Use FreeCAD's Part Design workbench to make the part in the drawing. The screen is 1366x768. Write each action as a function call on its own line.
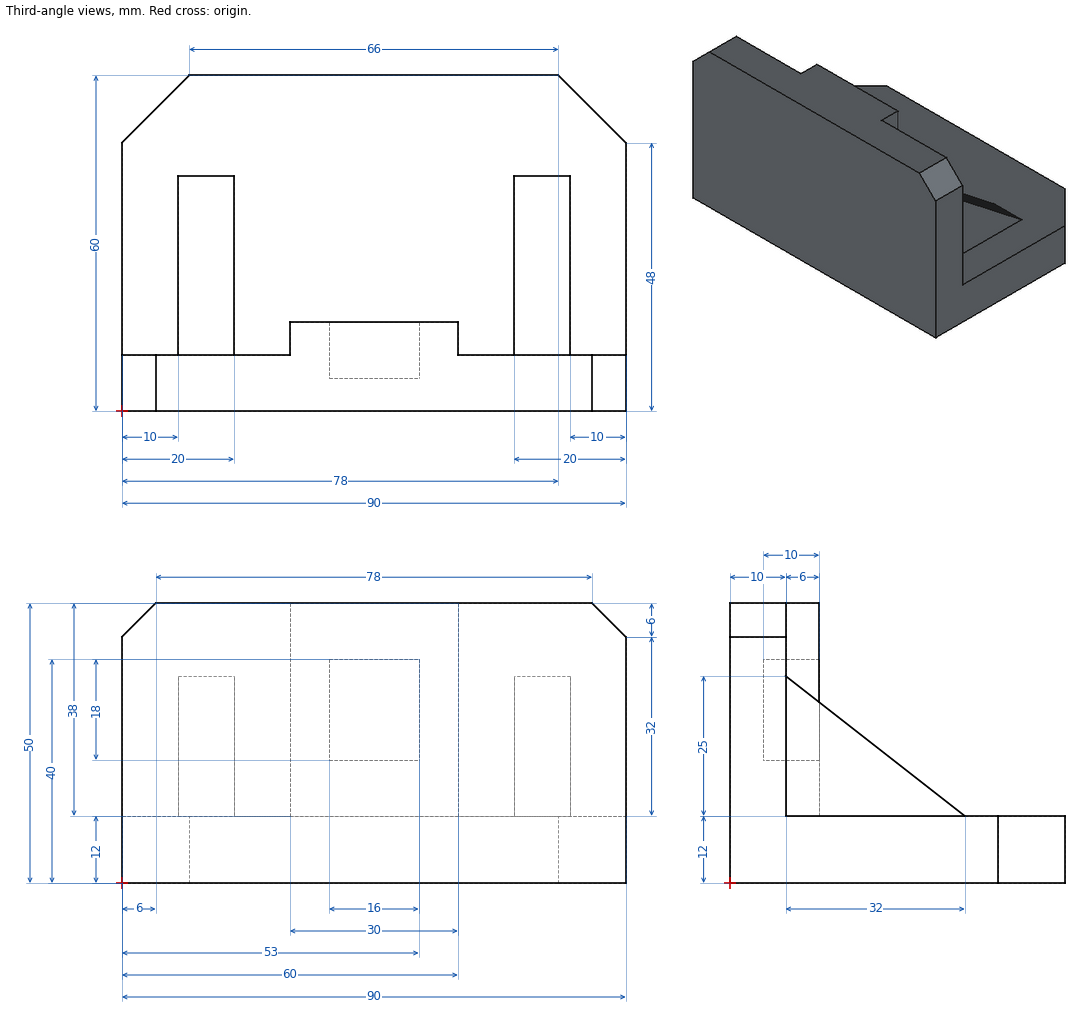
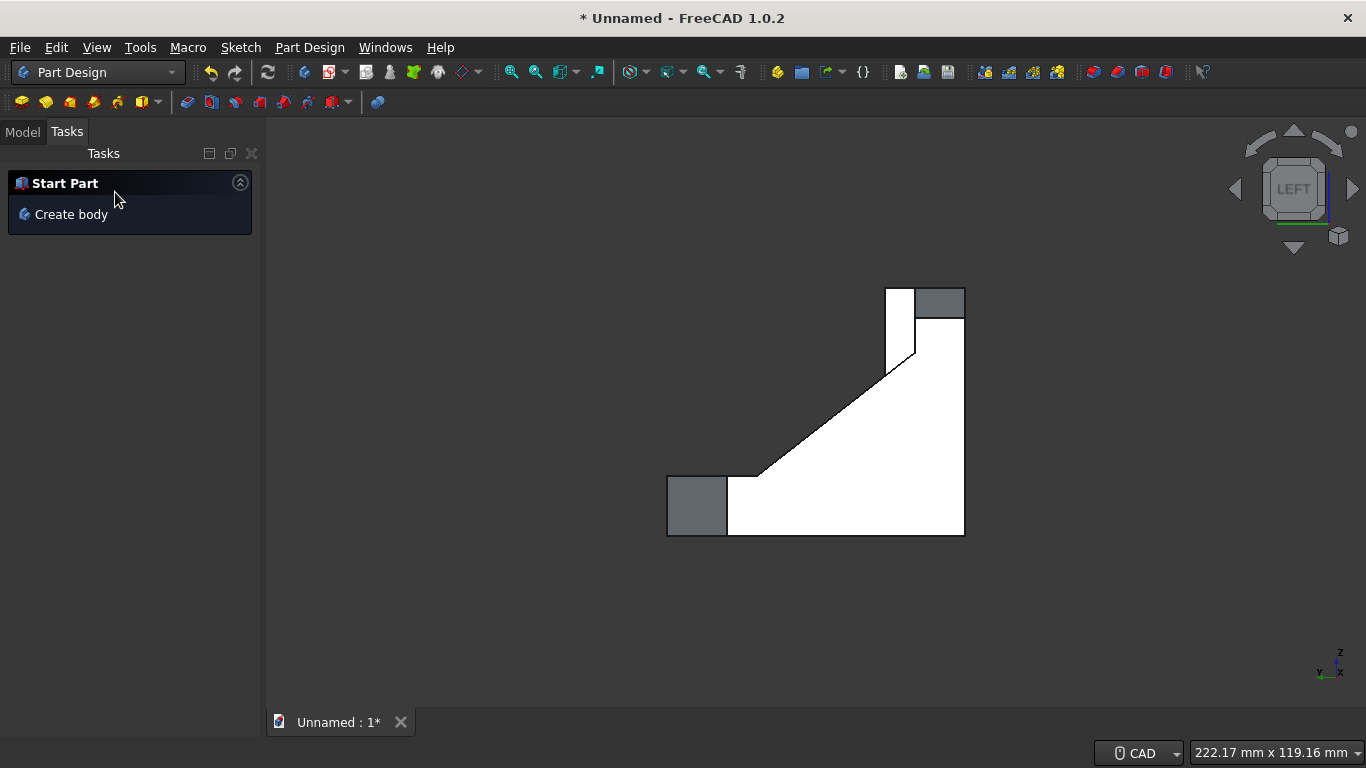
click(512, 72)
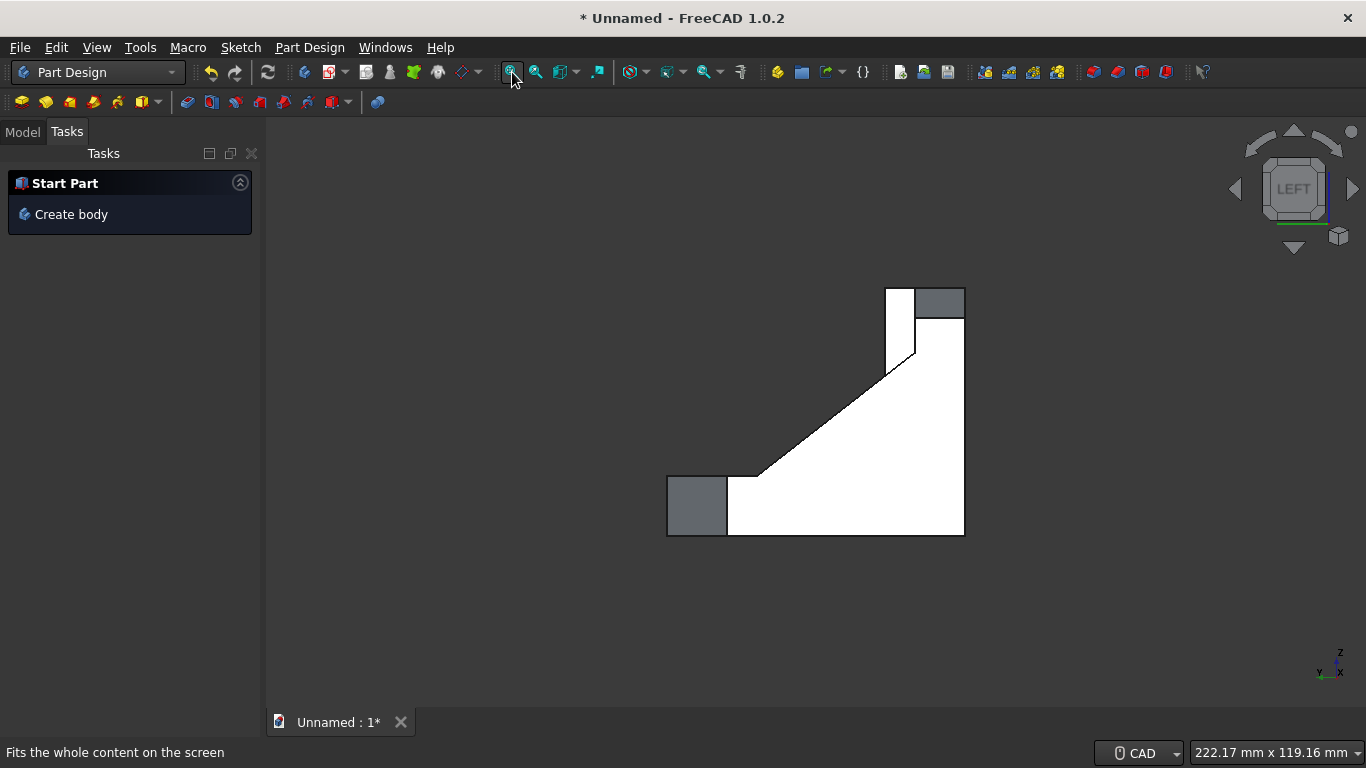
click(880, 457)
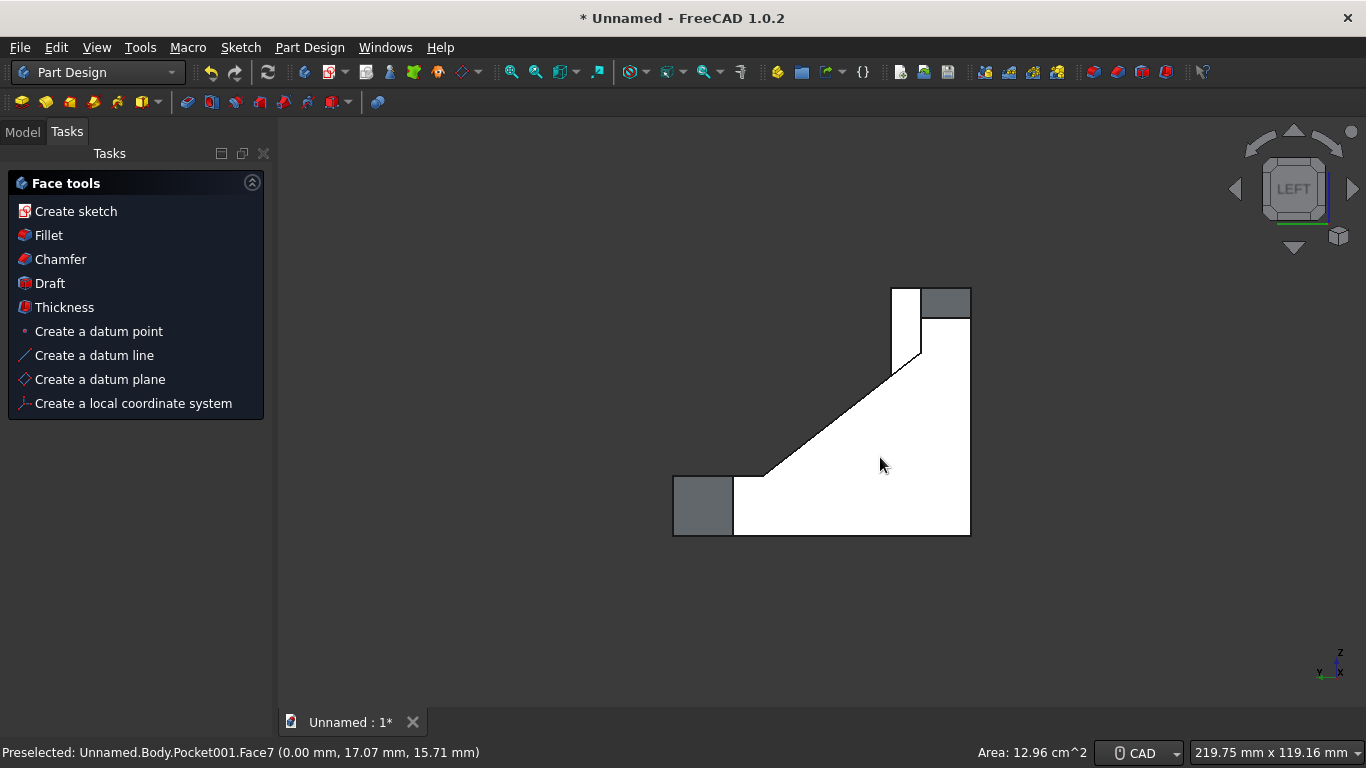
click(330, 72)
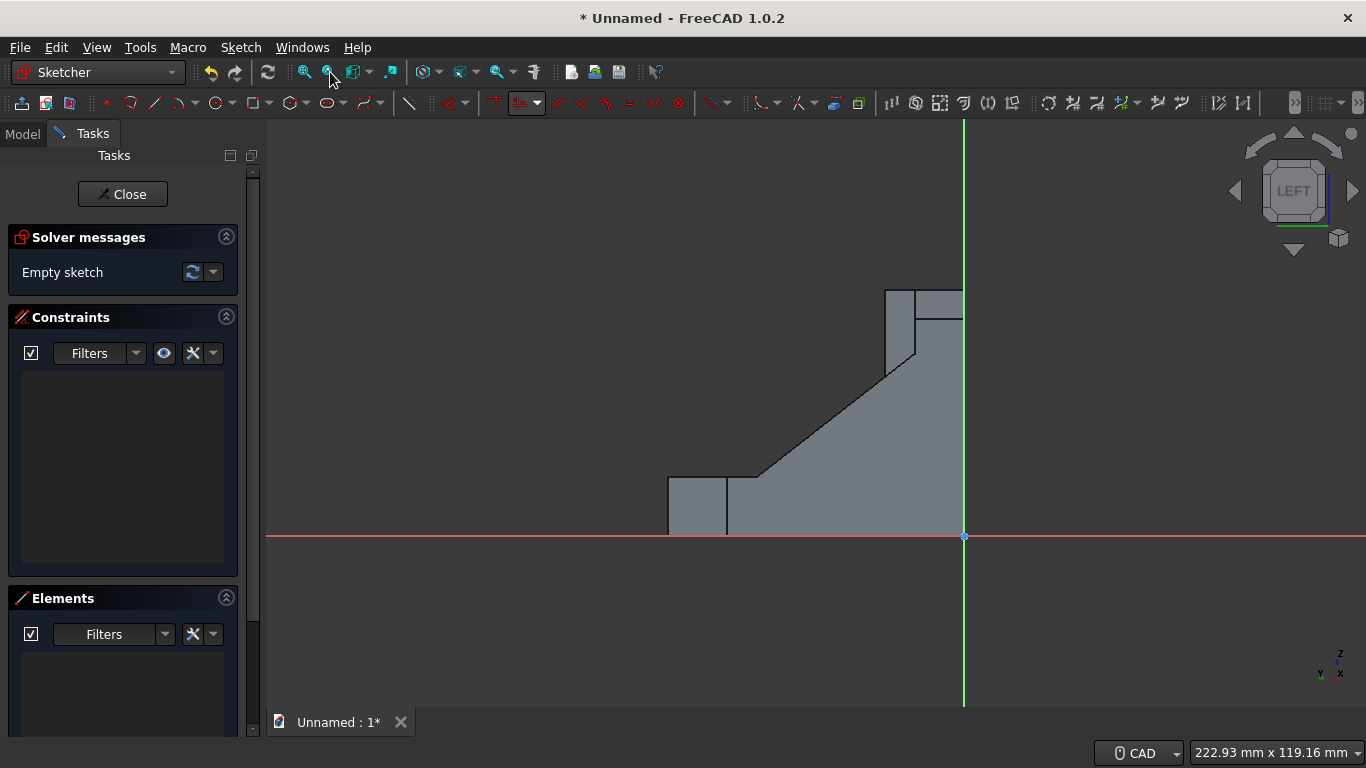
scroll(953, 471, up, 4)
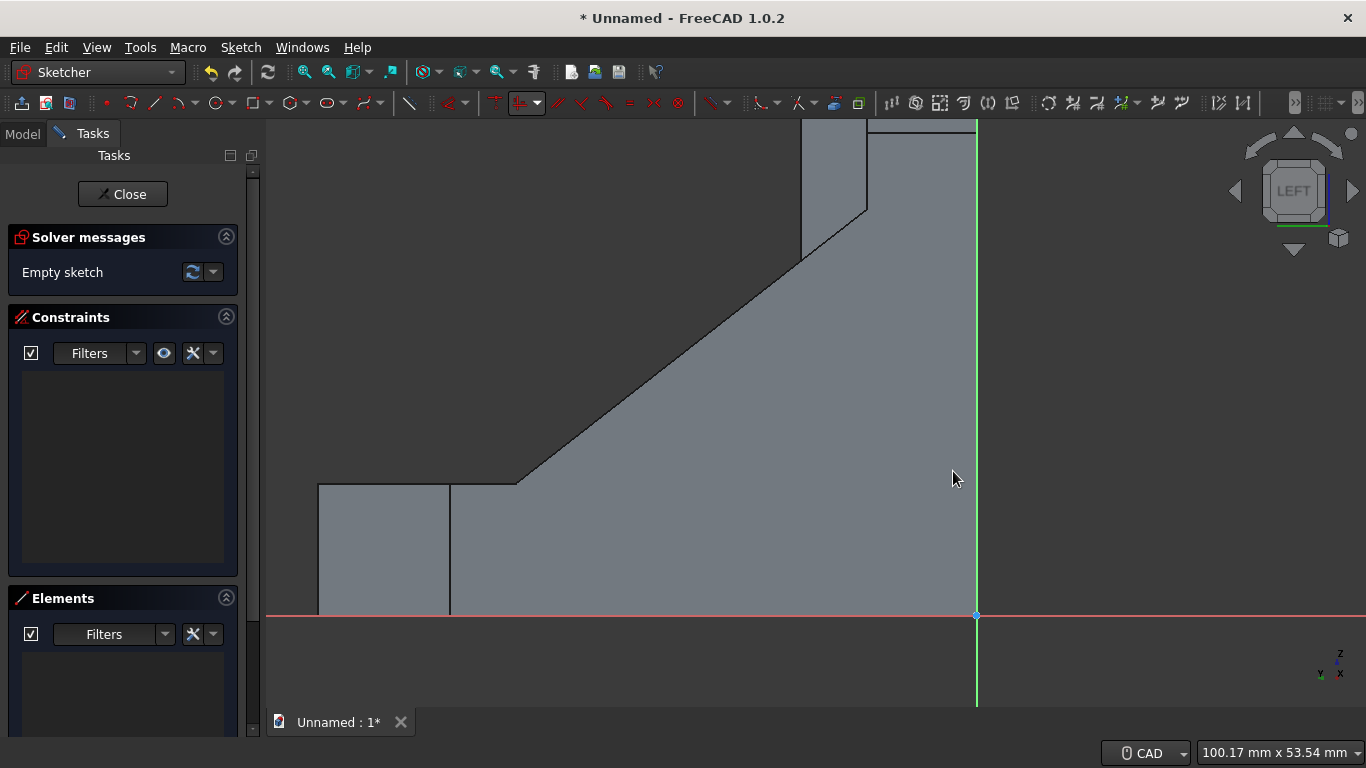
click(132, 104)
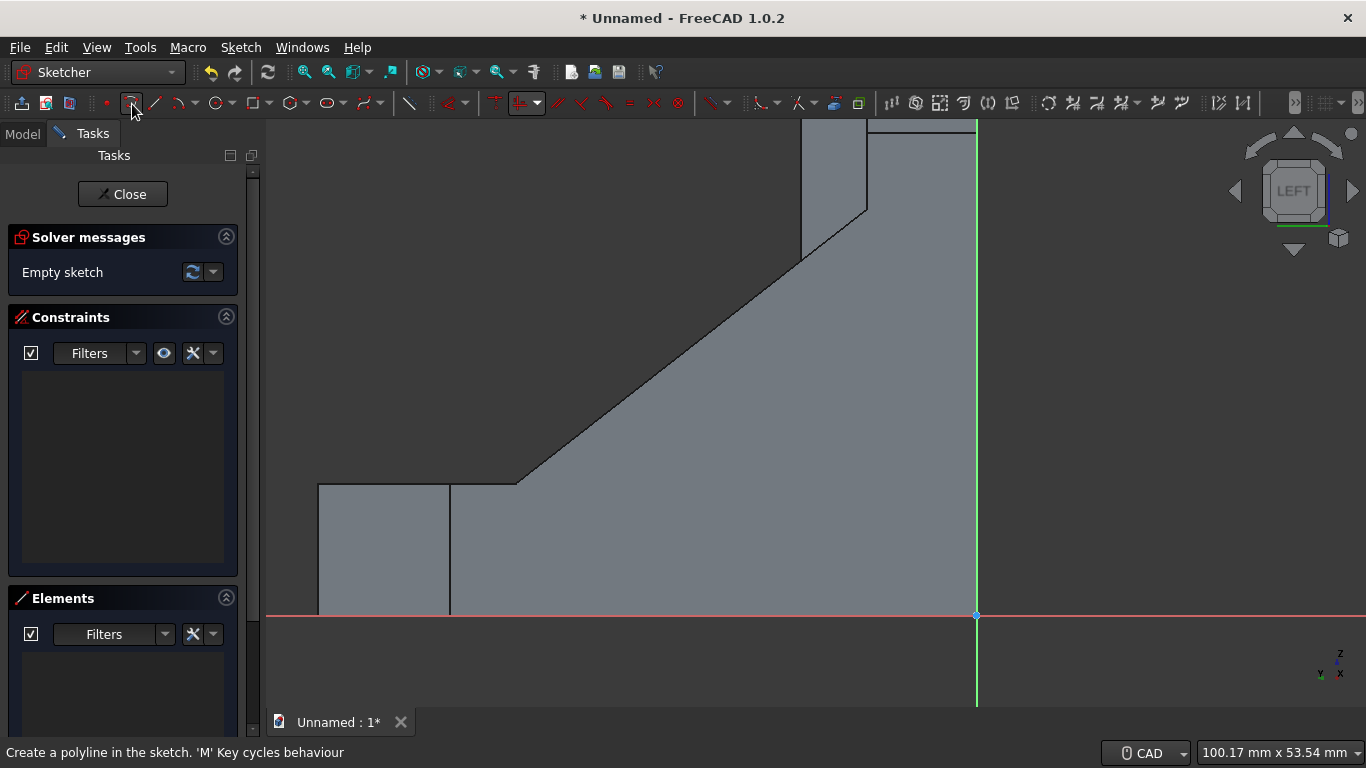
click(867, 484)
click(867, 209)
click(516, 484)
click(867, 485)
key(Escape)
key(Escape)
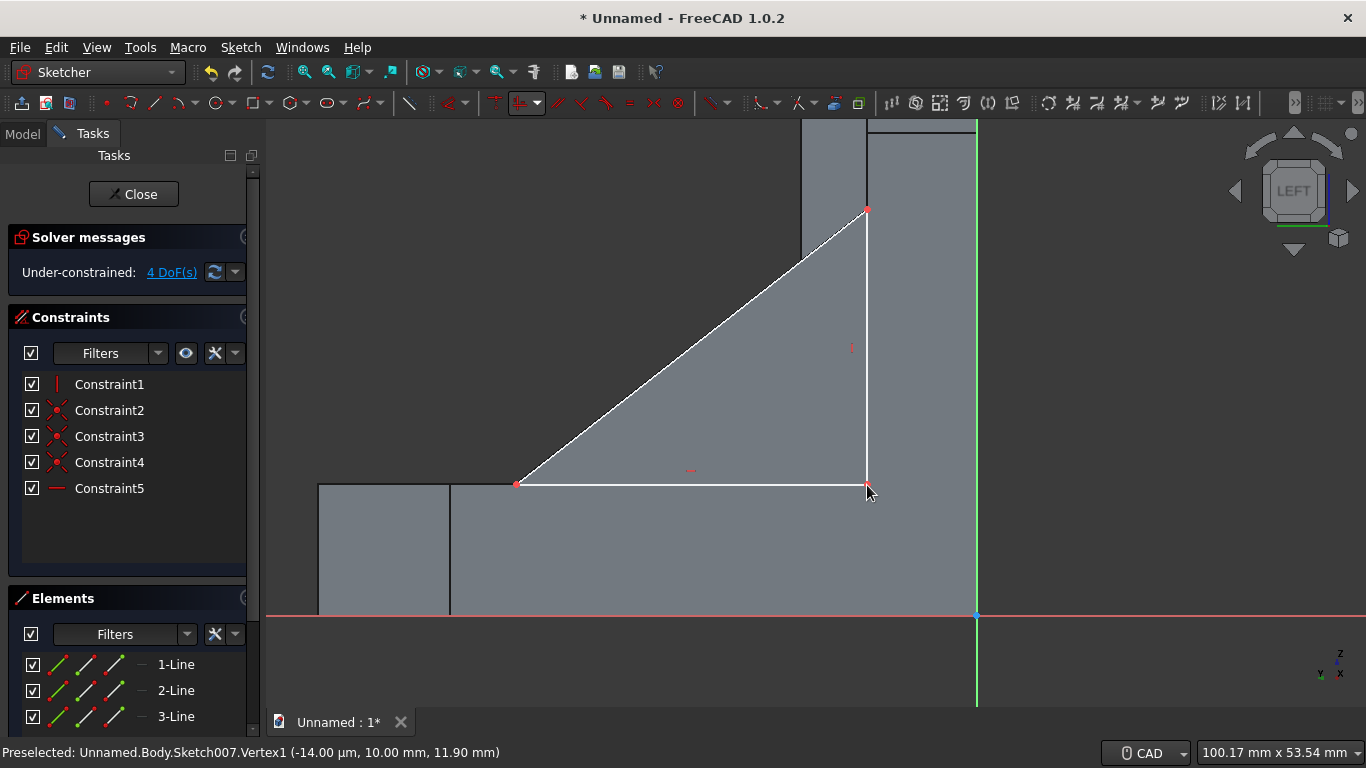
click(448, 104)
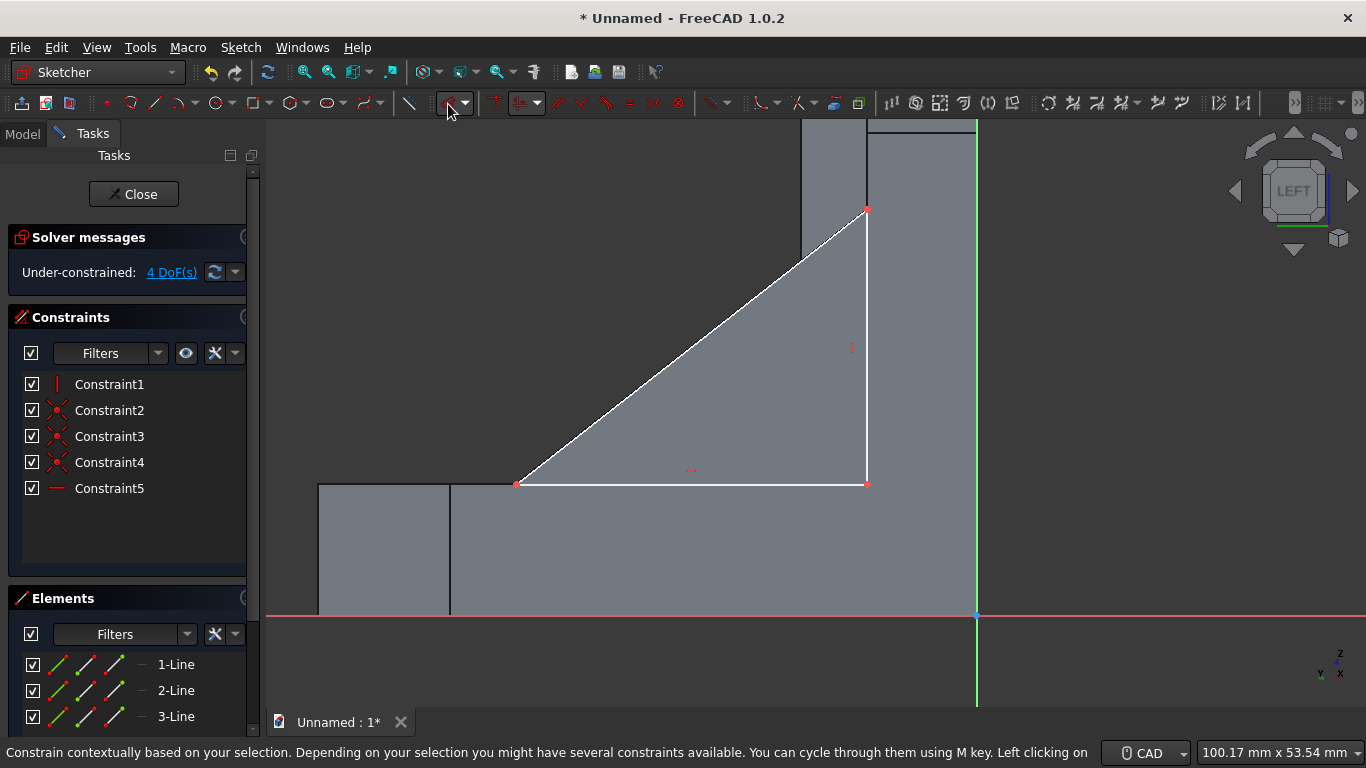
click(867, 403)
click(901, 347)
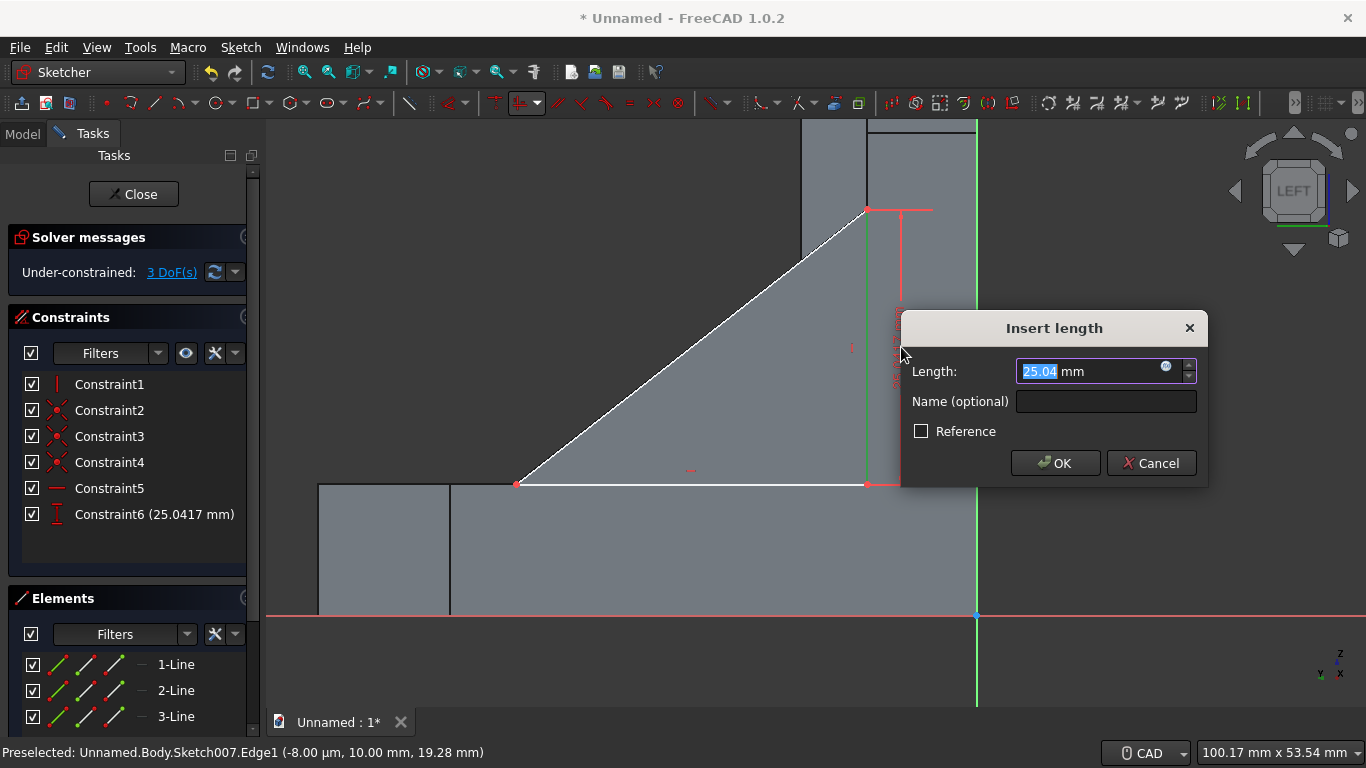
text(25)
key(Return)